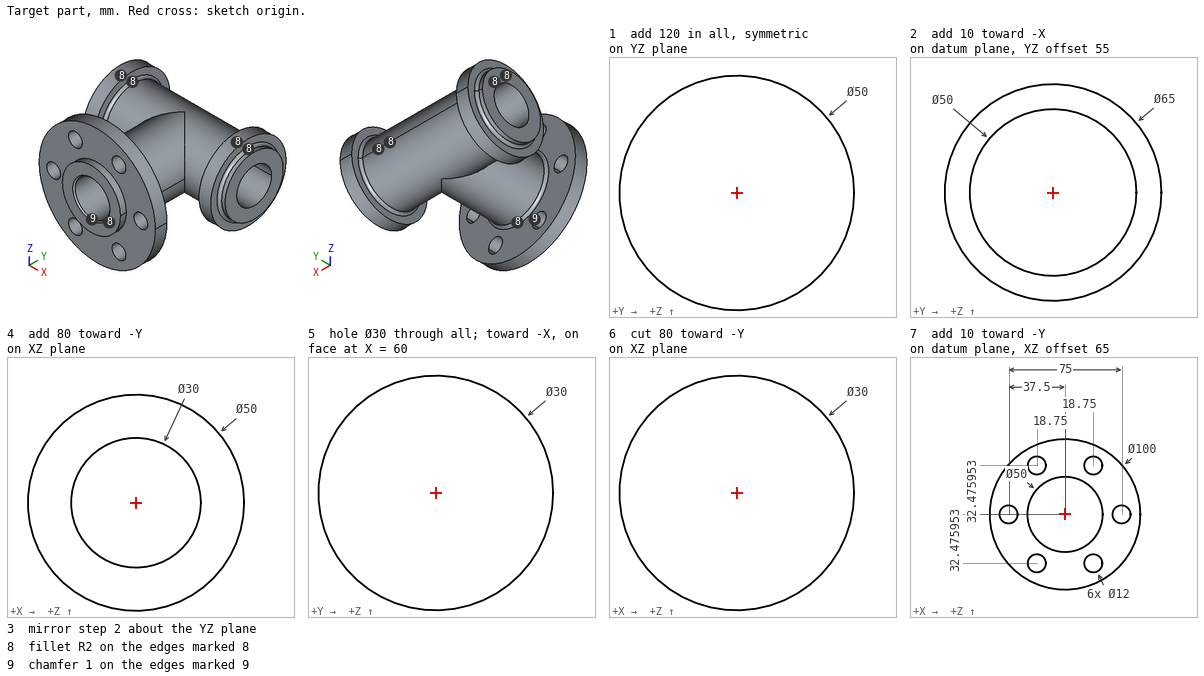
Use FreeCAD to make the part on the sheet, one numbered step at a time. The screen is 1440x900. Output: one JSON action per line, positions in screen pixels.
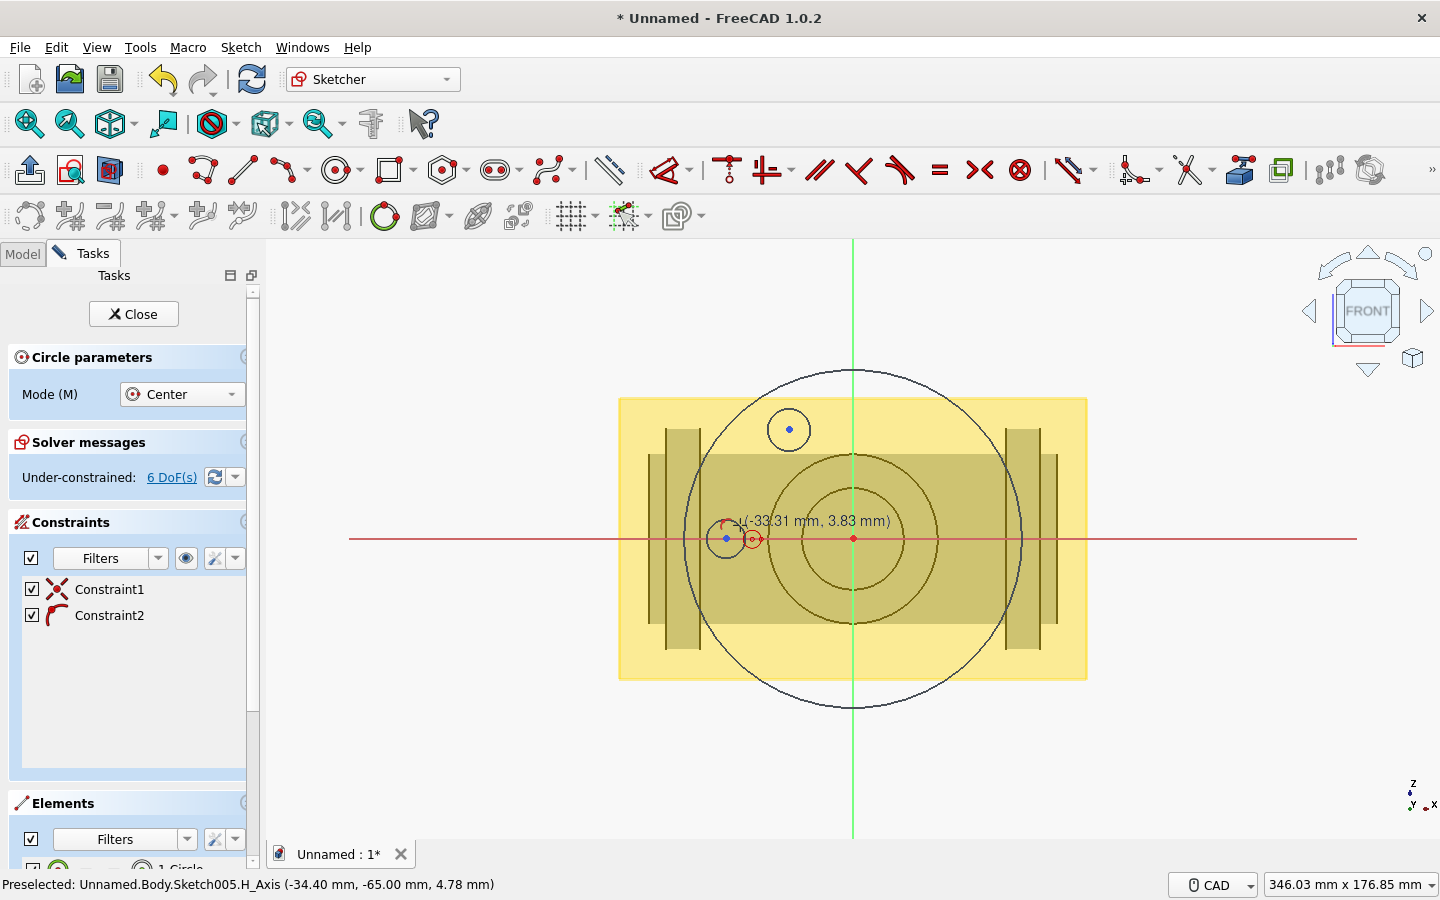
{"action": "left_click", "coordinate": [789, 649]}
{"action": "left_click", "coordinate": [804, 635]}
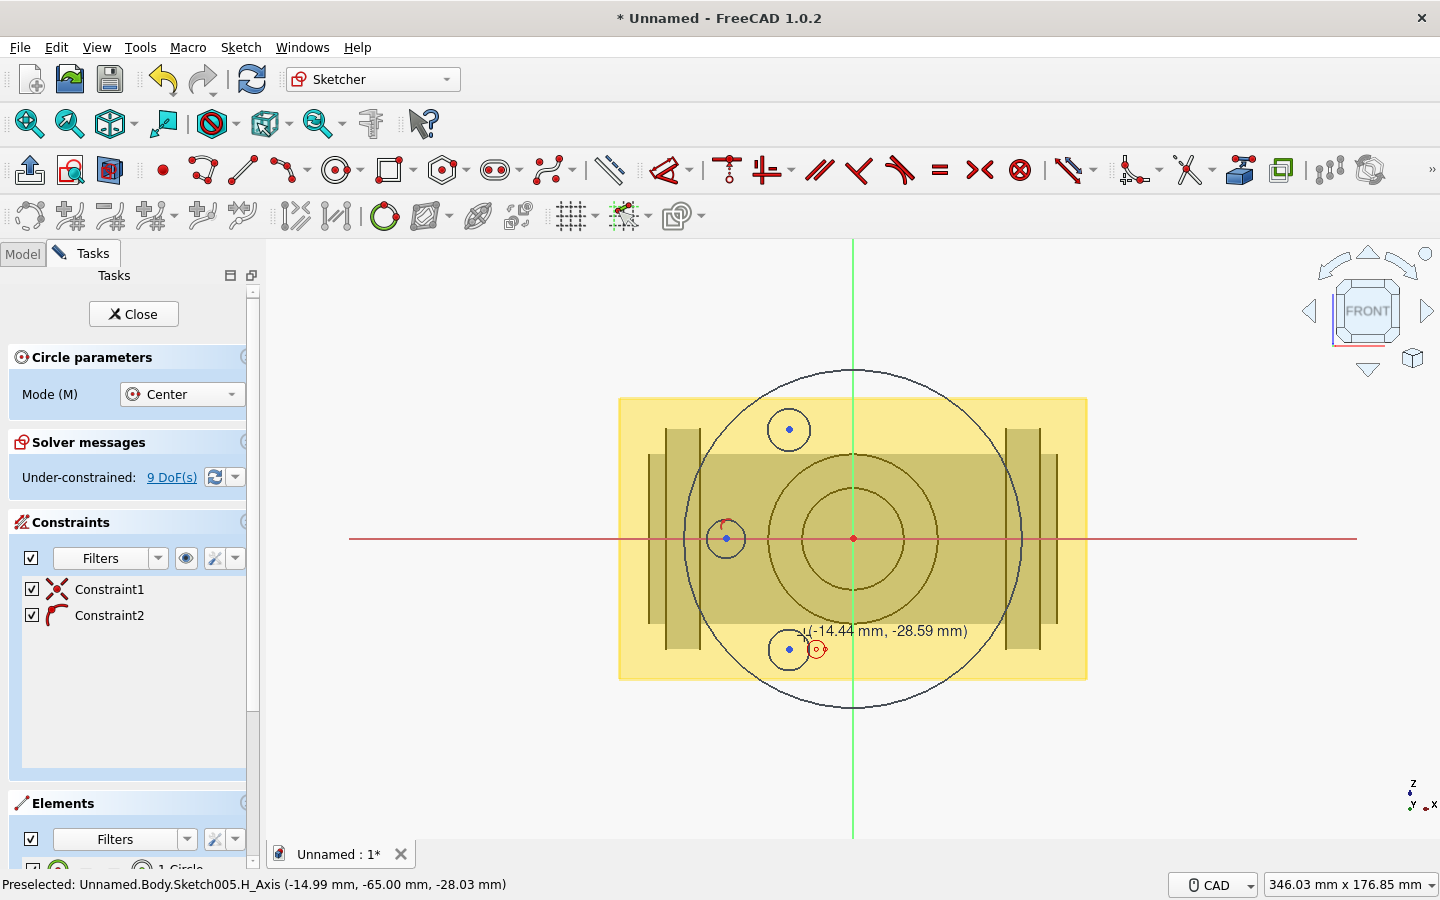
{"action": "left_click", "coordinate": [917, 429]}
{"action": "left_click", "coordinate": [931, 414]}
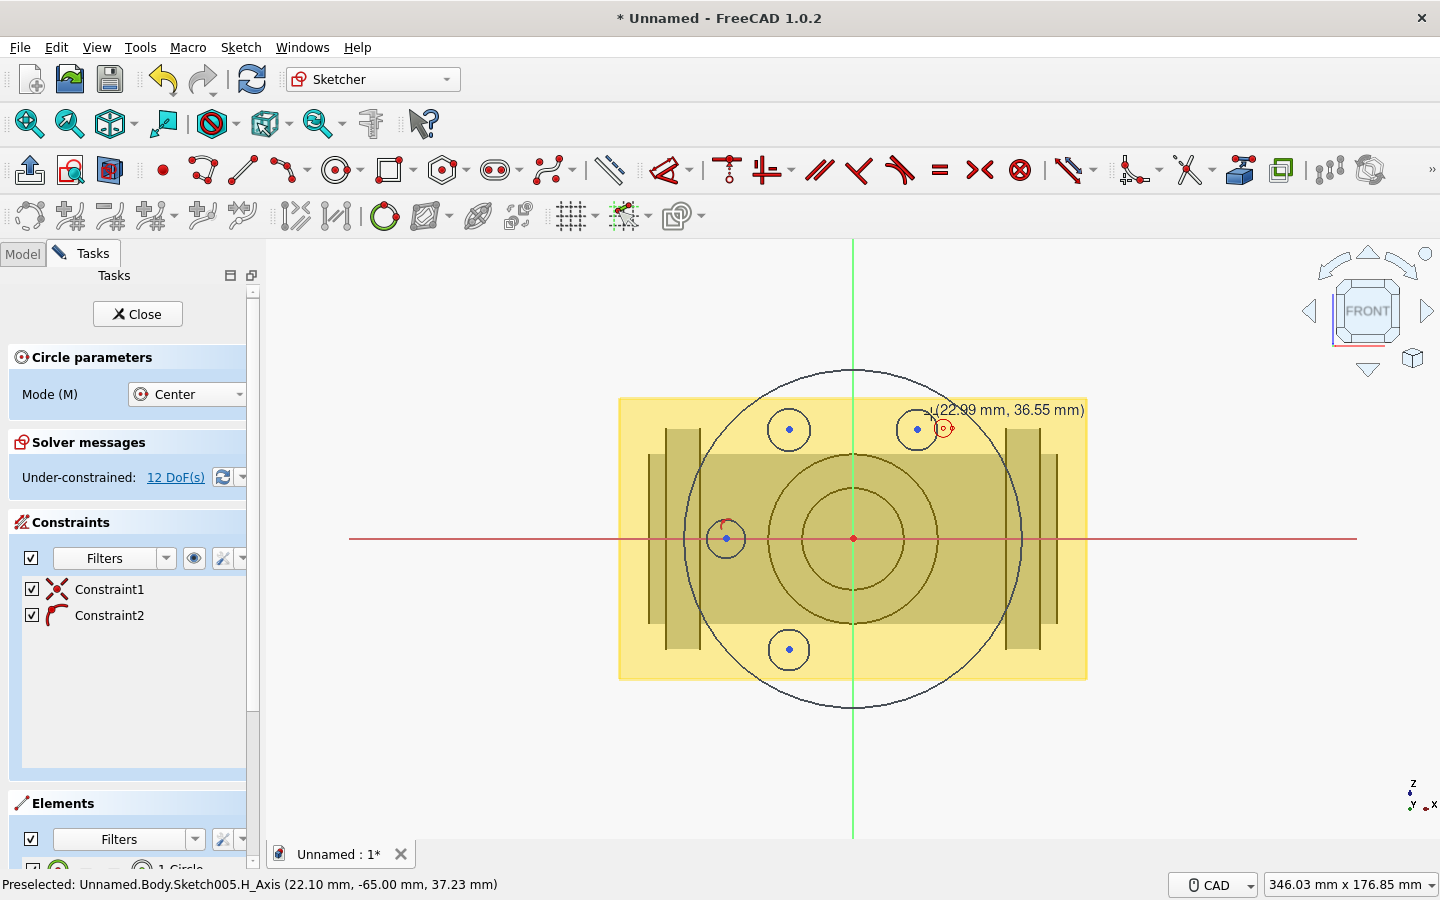
{"action": "left_click", "coordinate": [980, 539]}
{"action": "left_click", "coordinate": [995, 525]}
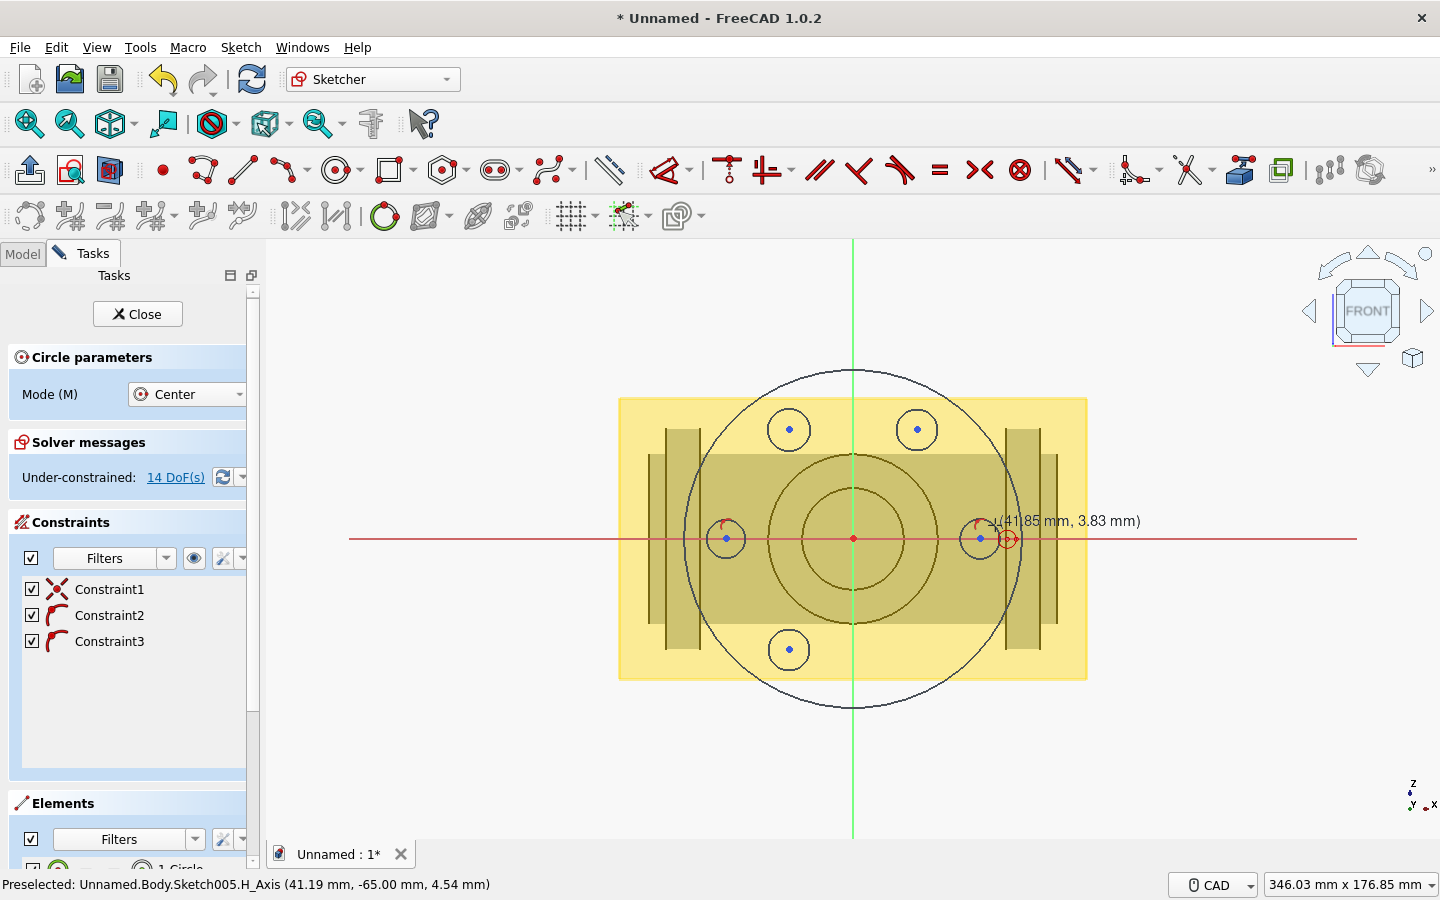
{"action": "left_click", "coordinate": [853, 539]}
{"action": "left_click", "coordinate": [913, 479]}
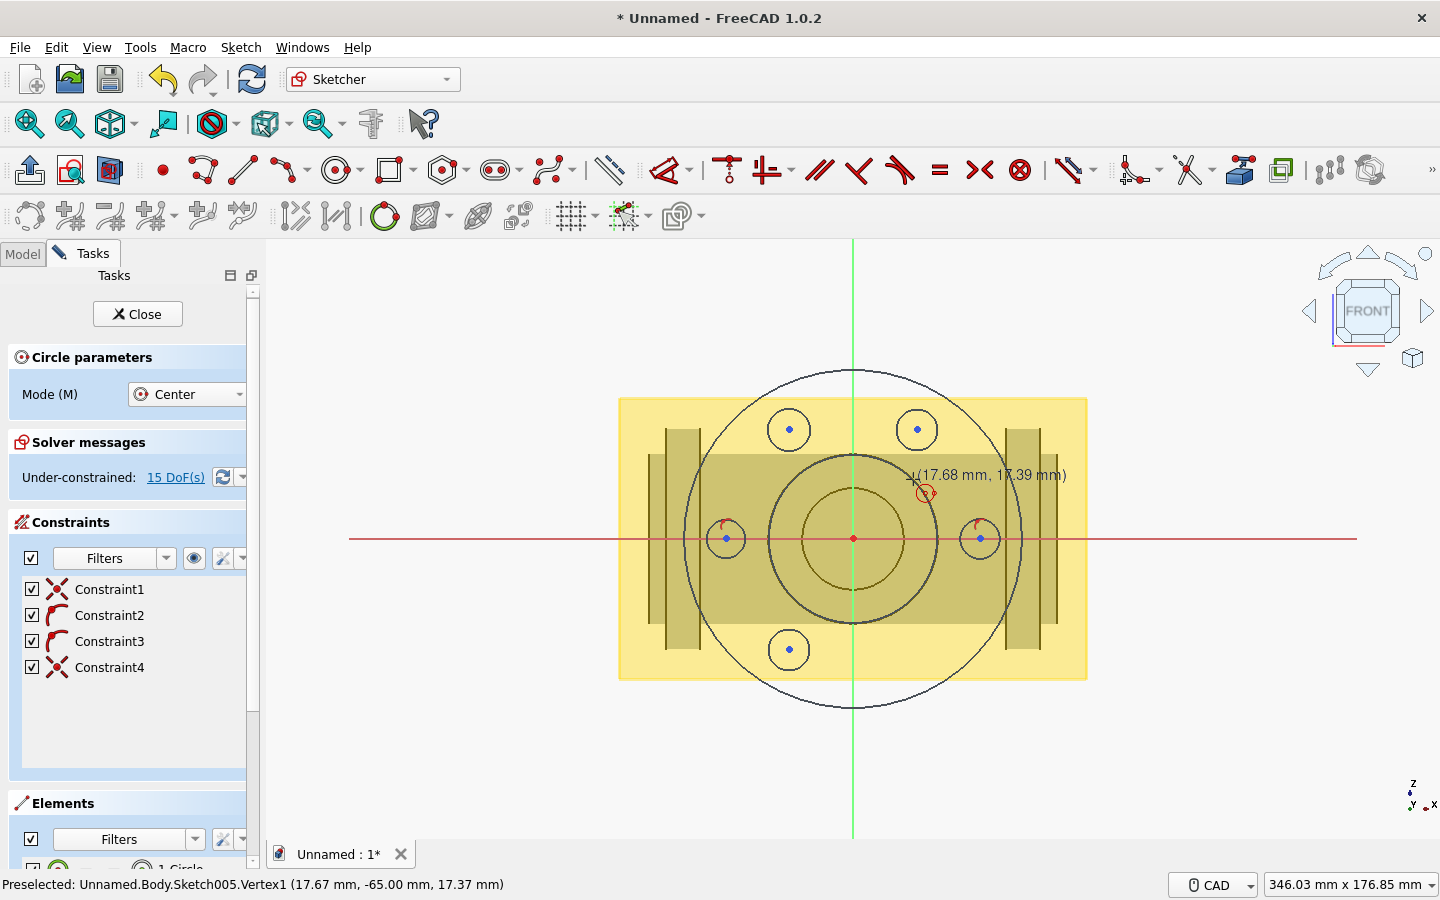
{"action": "left_click", "coordinate": [917, 649]}
{"action": "left_click", "coordinate": [931, 635]}
{"action": "key", "text": "Escape"}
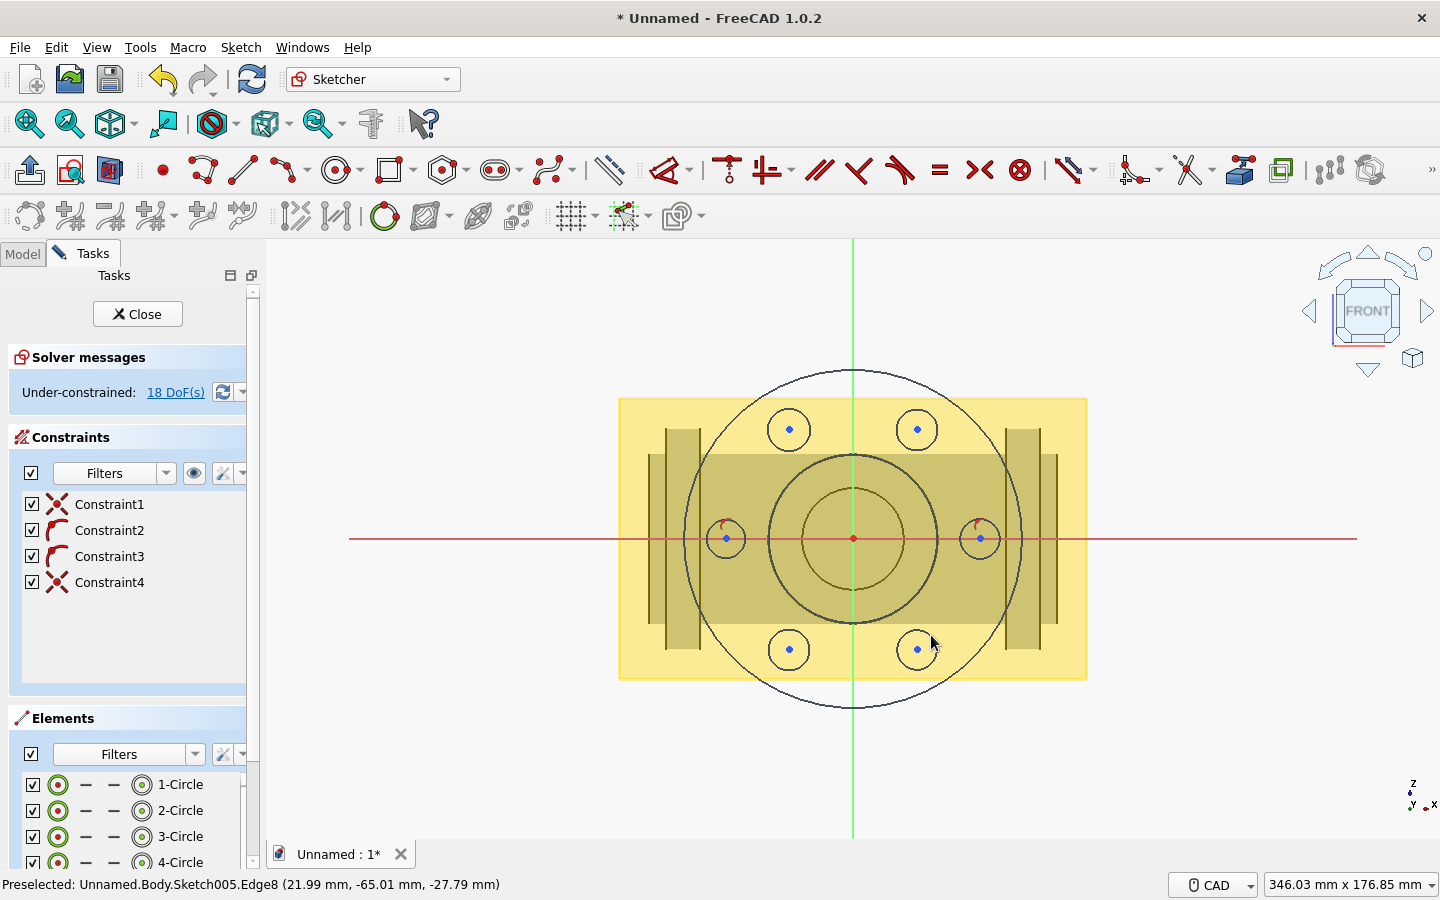
{"action": "left_click", "coordinate": [804, 415]}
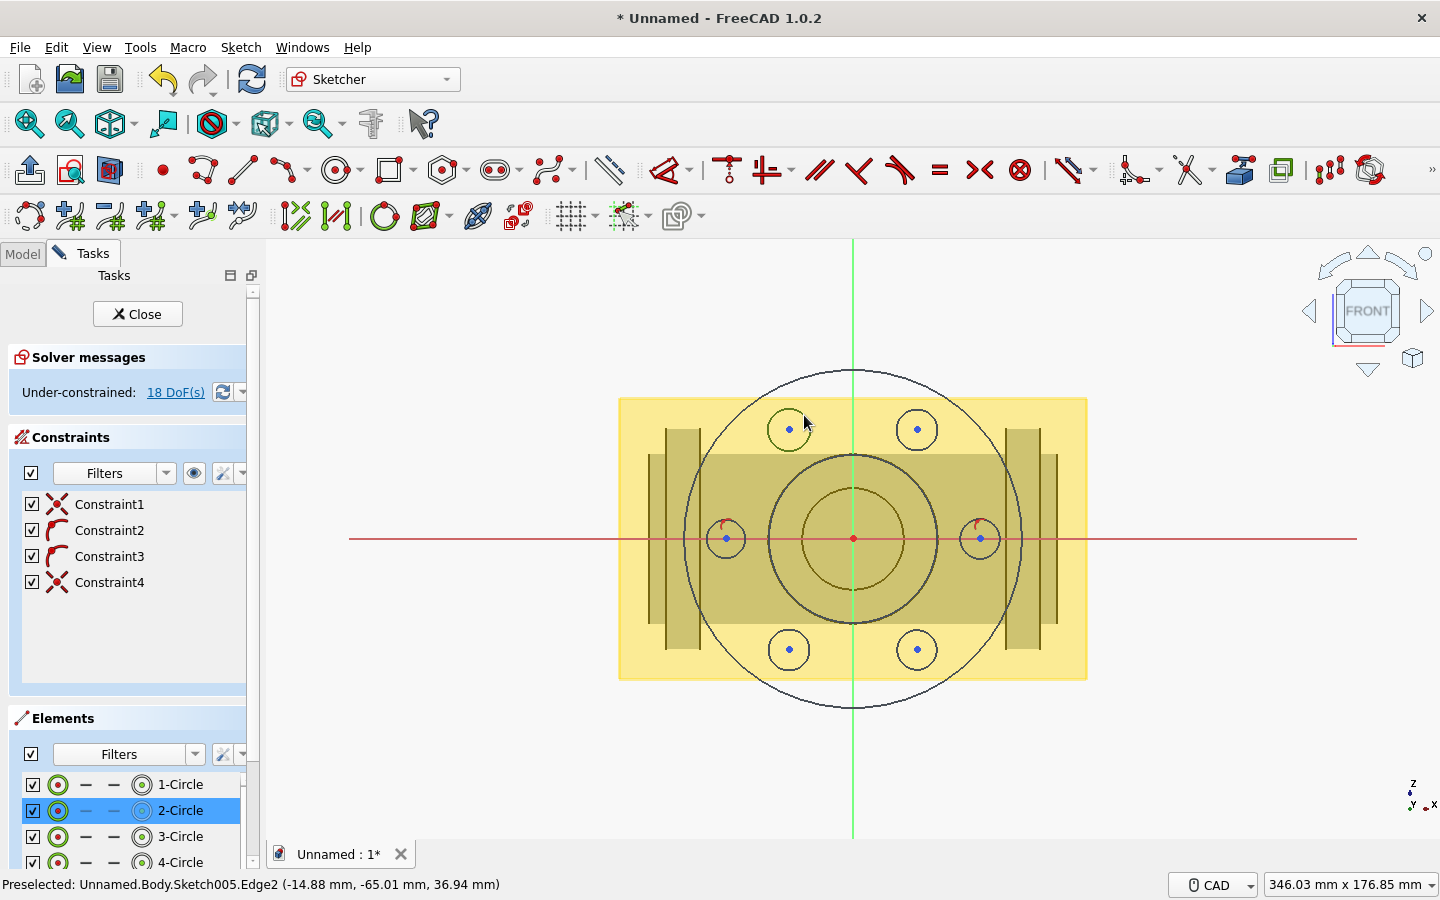
{"action": "left_click", "coordinate": [739, 525]}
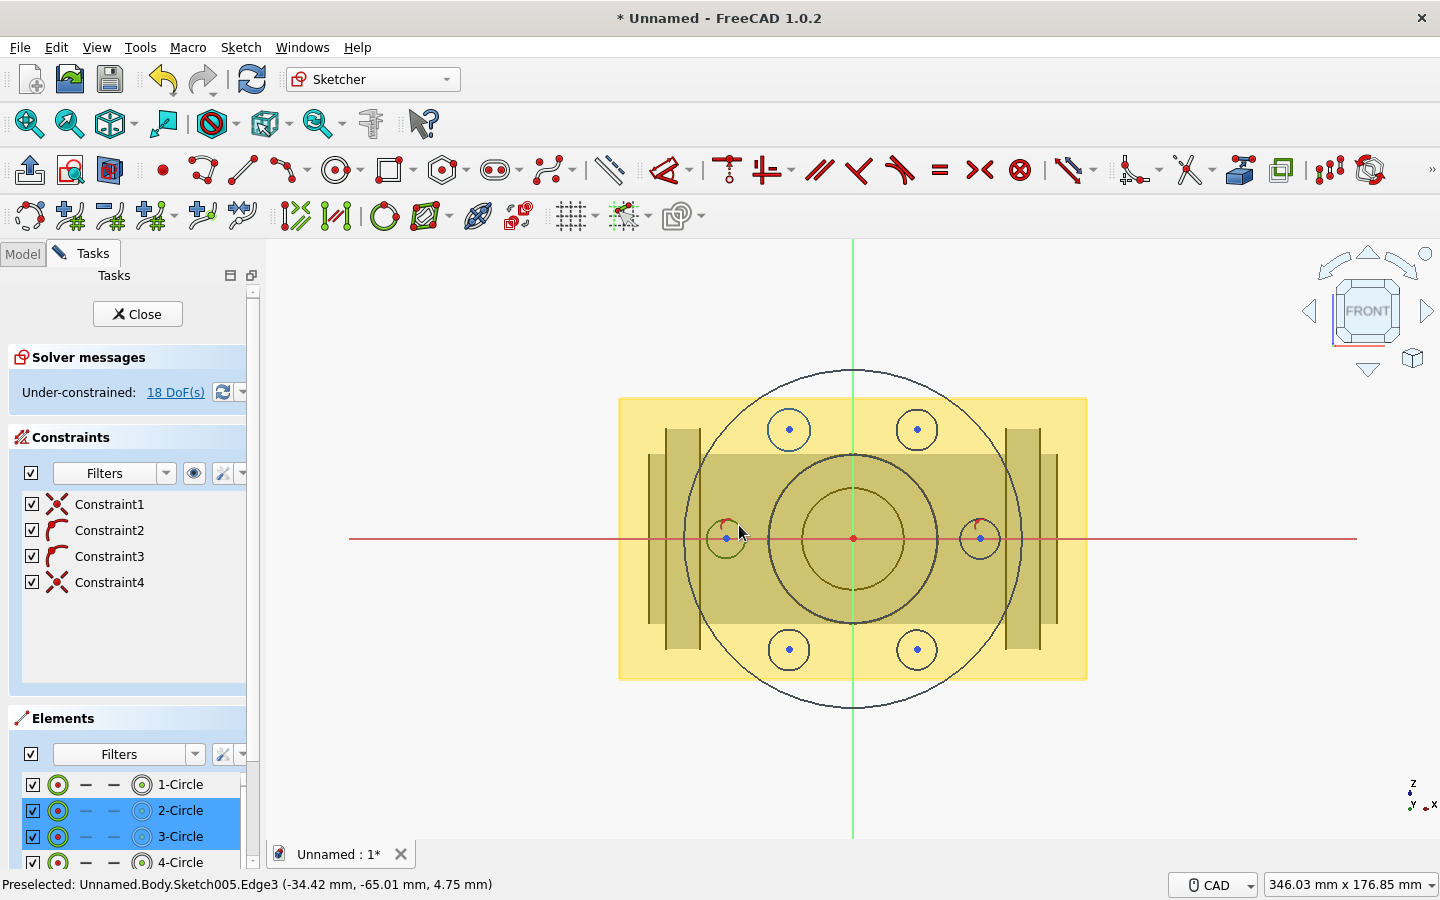
{"action": "left_click", "coordinate": [803, 635]}